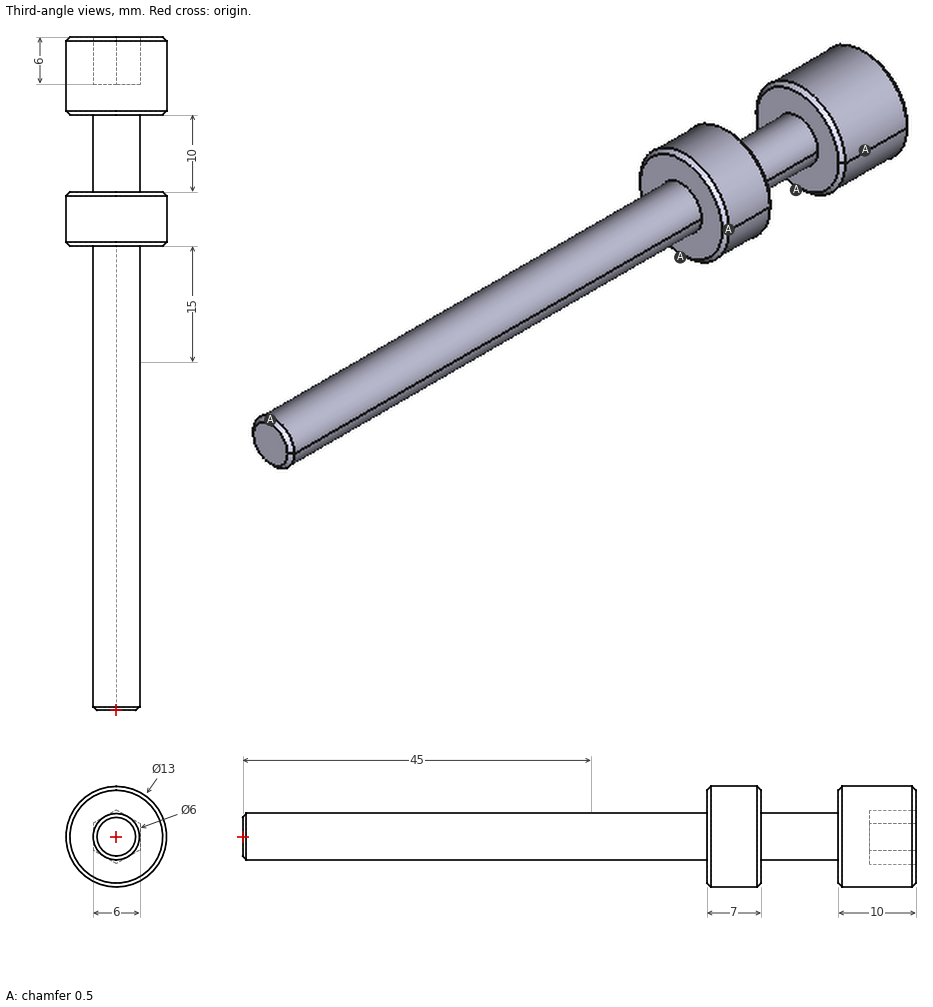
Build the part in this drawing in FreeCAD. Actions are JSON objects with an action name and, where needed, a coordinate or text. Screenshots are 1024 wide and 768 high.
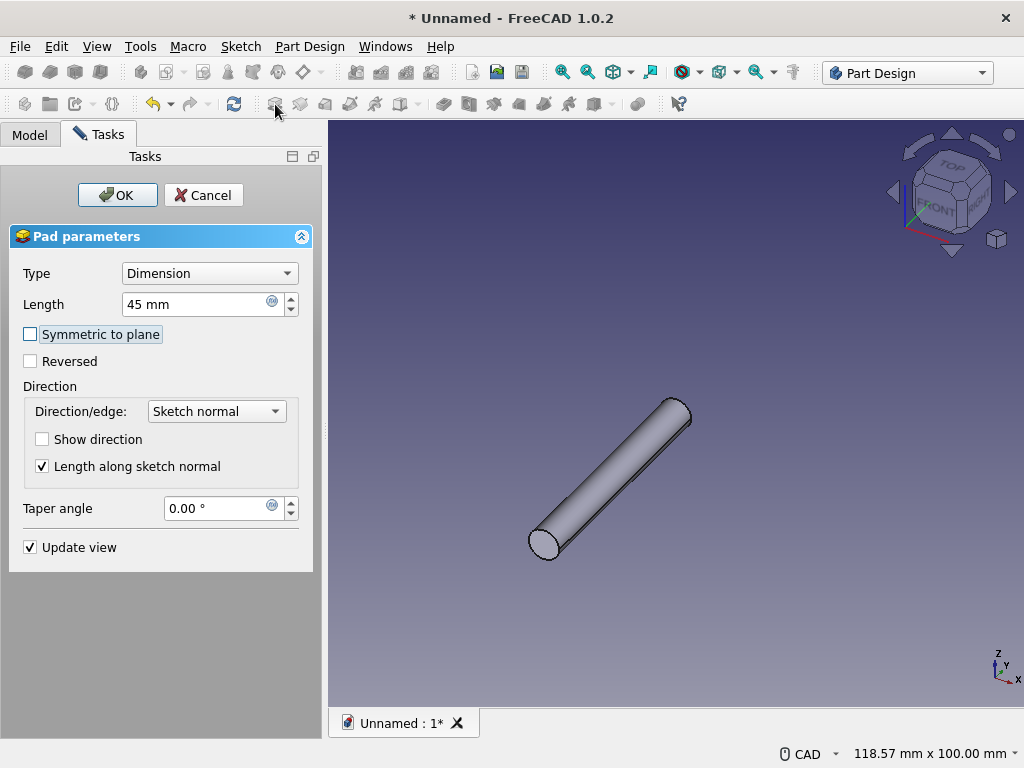
{"action": "left_click", "coordinate": [31, 361]}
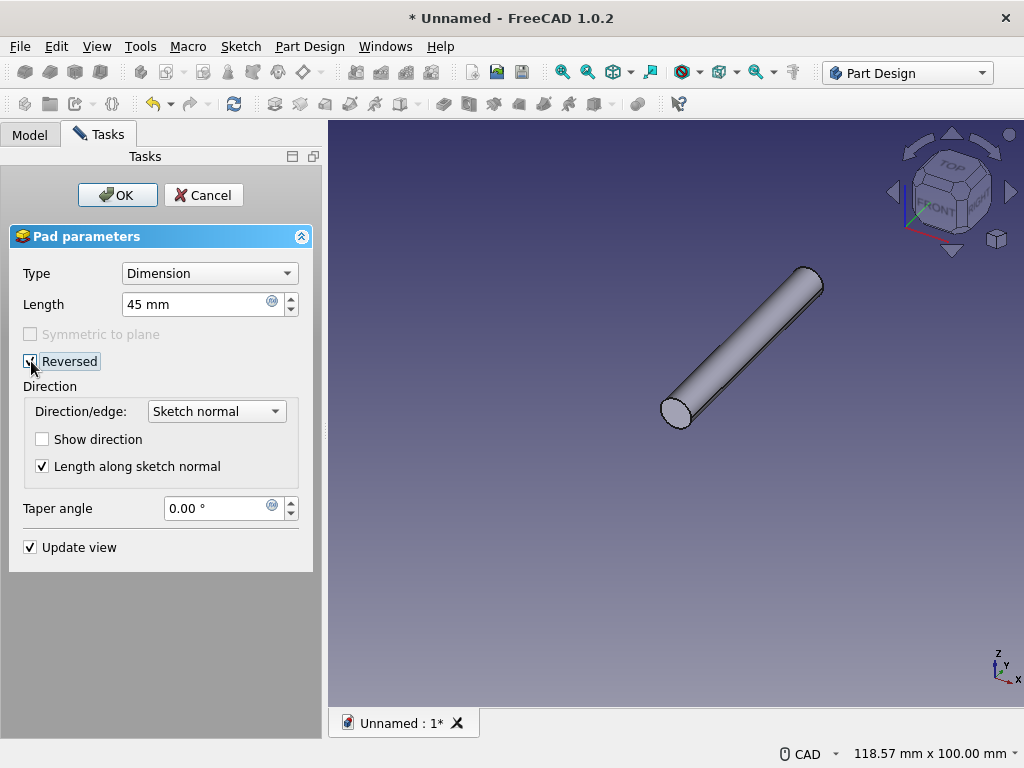
{"action": "left_click", "coordinate": [118, 195]}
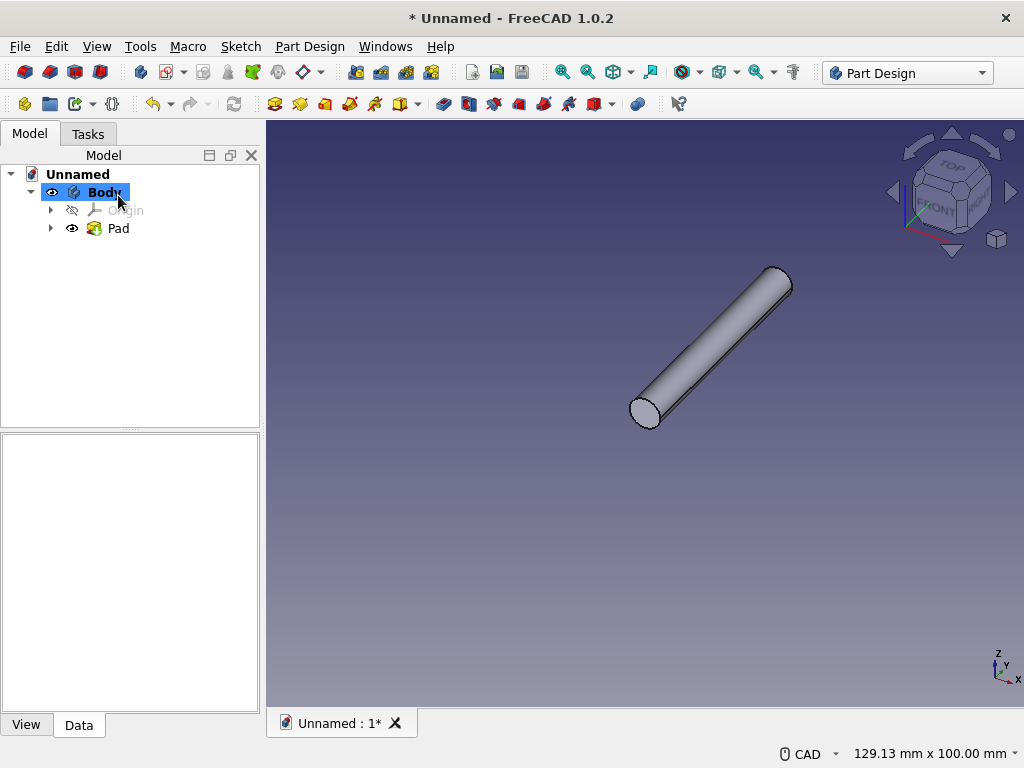
{"action": "left_click", "coordinate": [563, 72]}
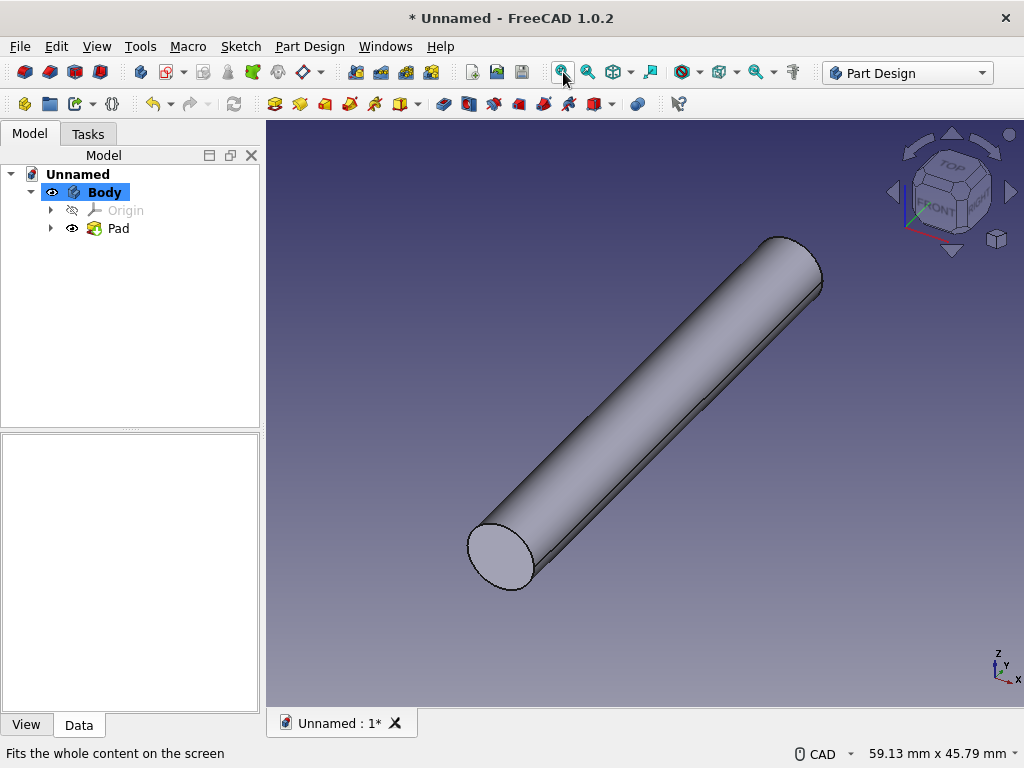
{"action": "key", "text": "4"}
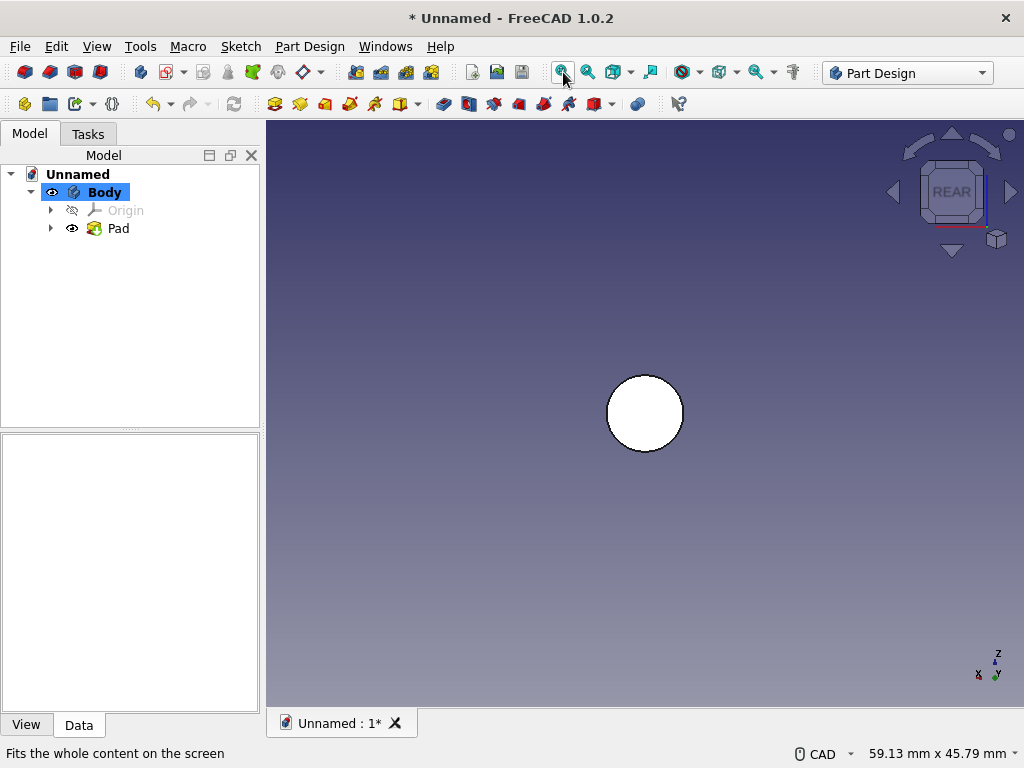
{"action": "left_click", "coordinate": [563, 72]}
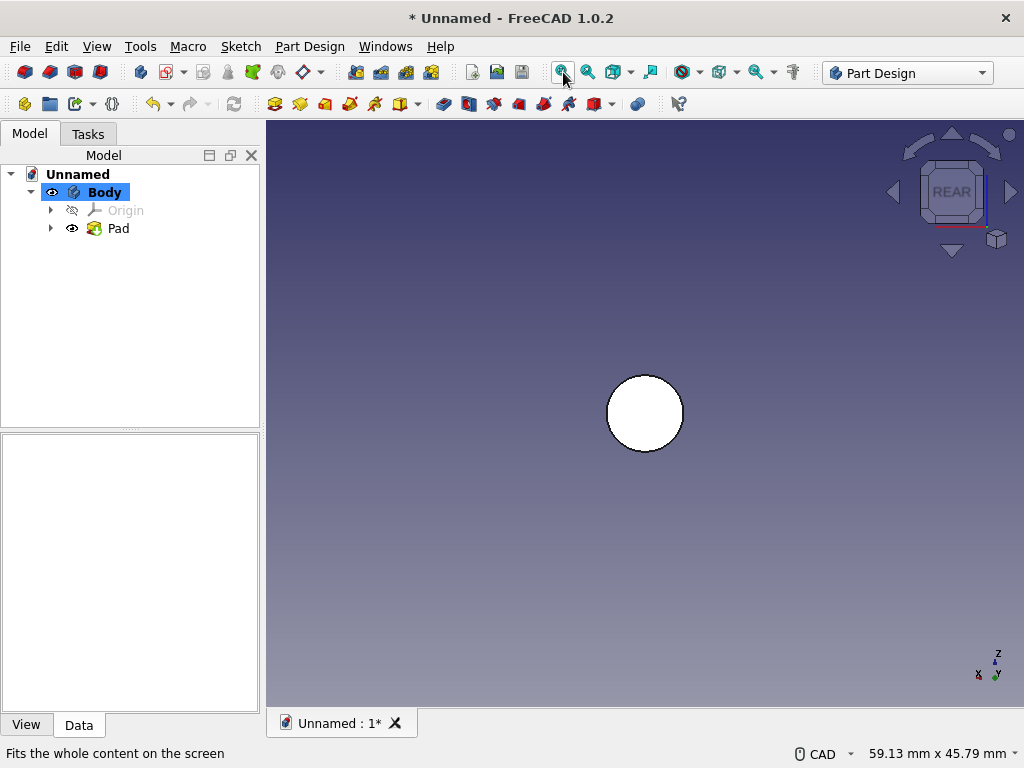
{"action": "left_click", "coordinate": [645, 413]}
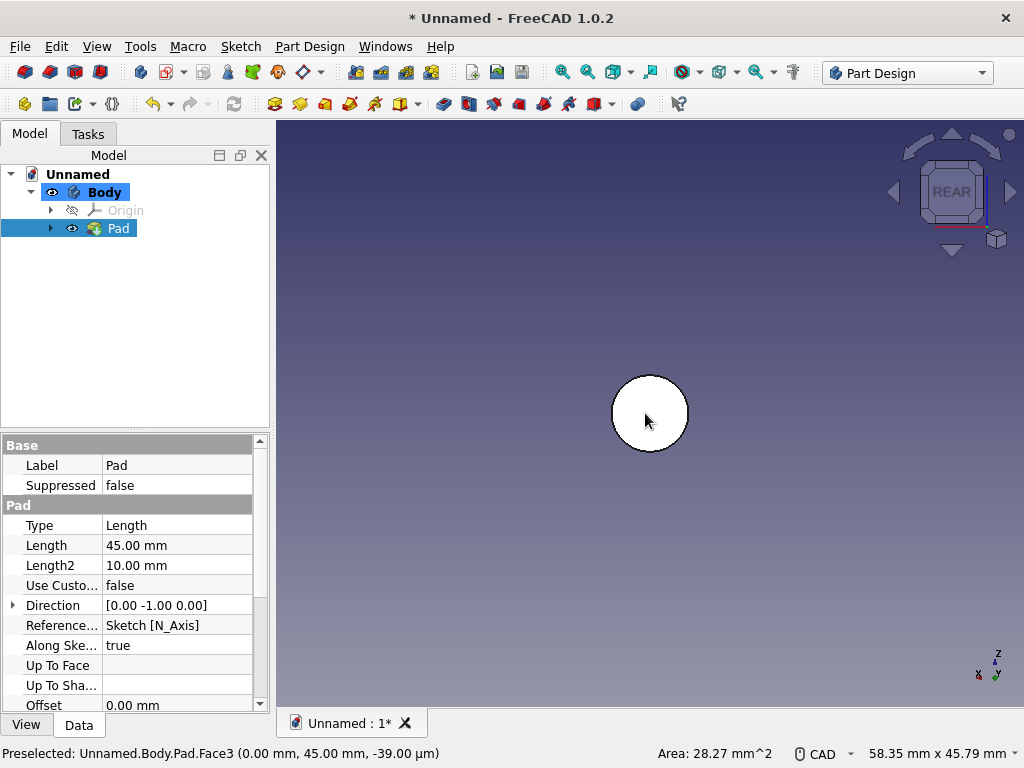
{"action": "left_click", "coordinate": [166, 72]}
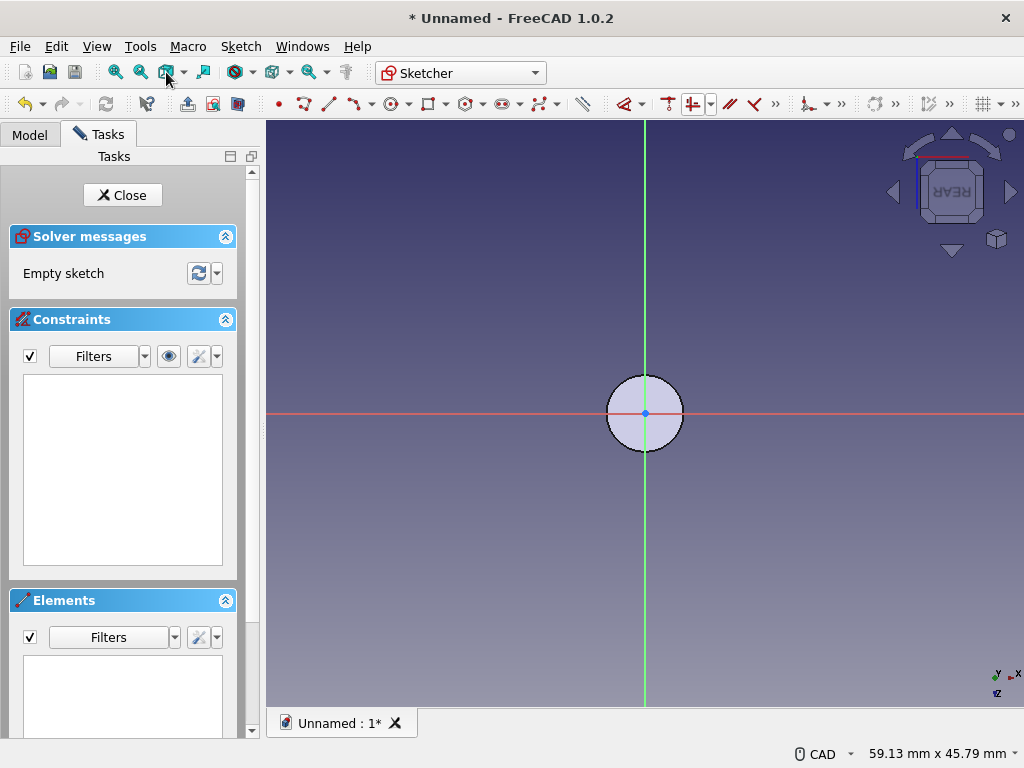
{"action": "scroll", "coordinate": [662, 413], "scroll_direction": "up", "scroll_amount": 8}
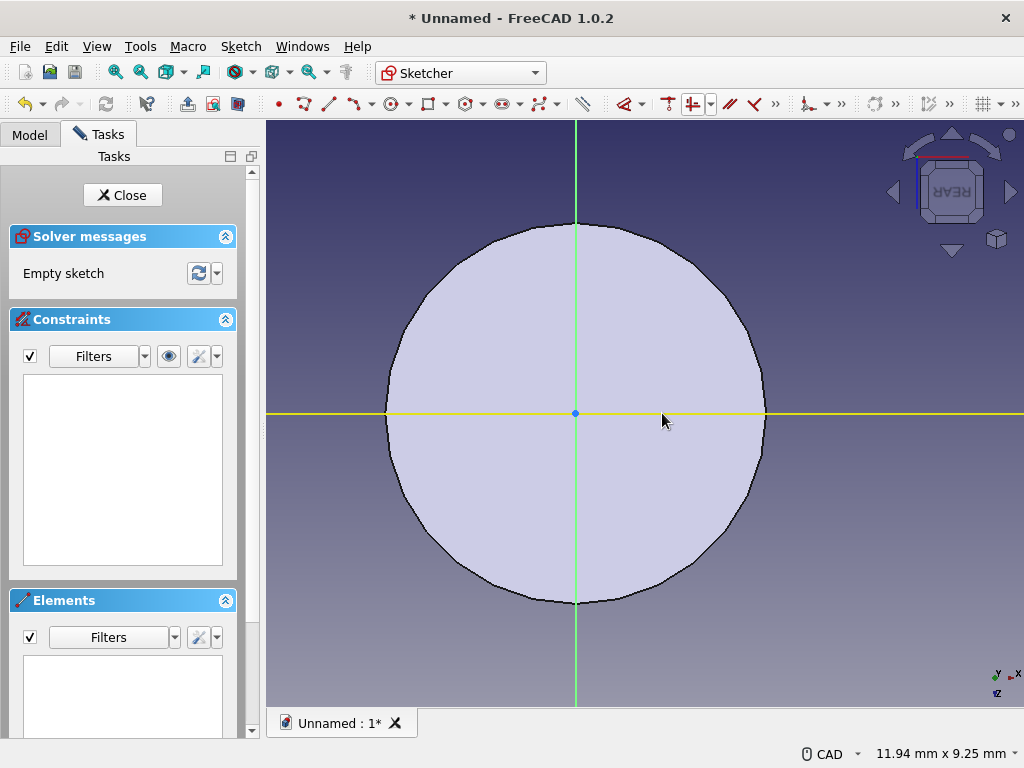
{"action": "left_click", "coordinate": [390, 104]}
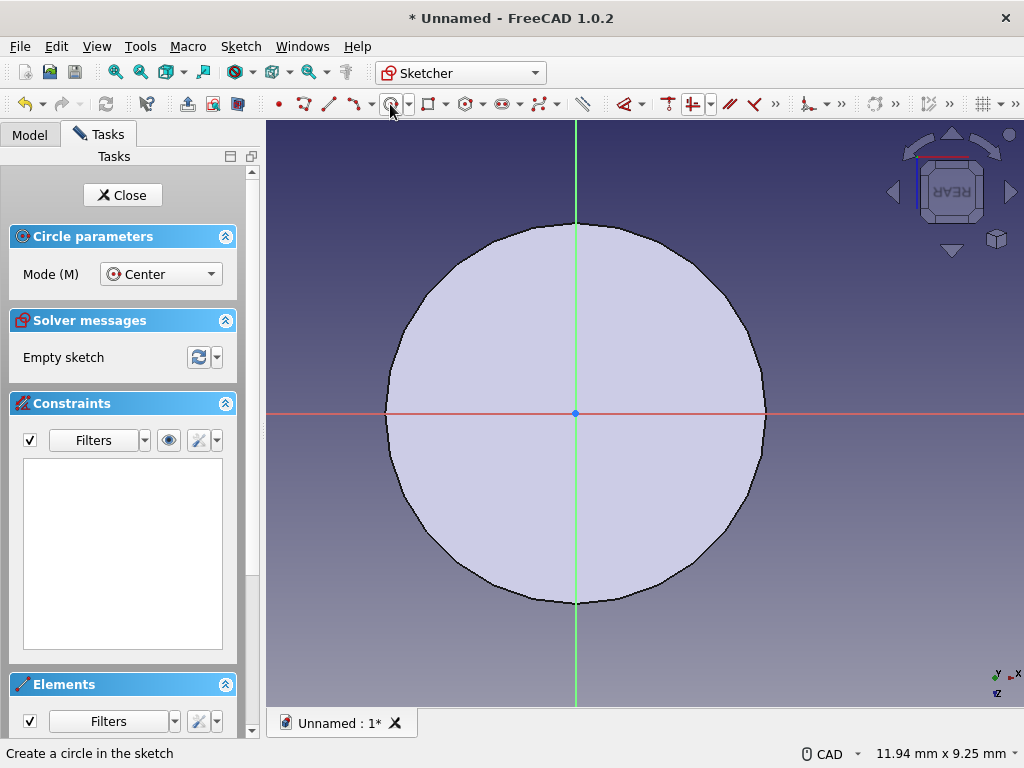
{"action": "left_click", "coordinate": [576, 413]}
{"action": "left_click", "coordinate": [710, 279]}
{"action": "key", "text": "Escape"}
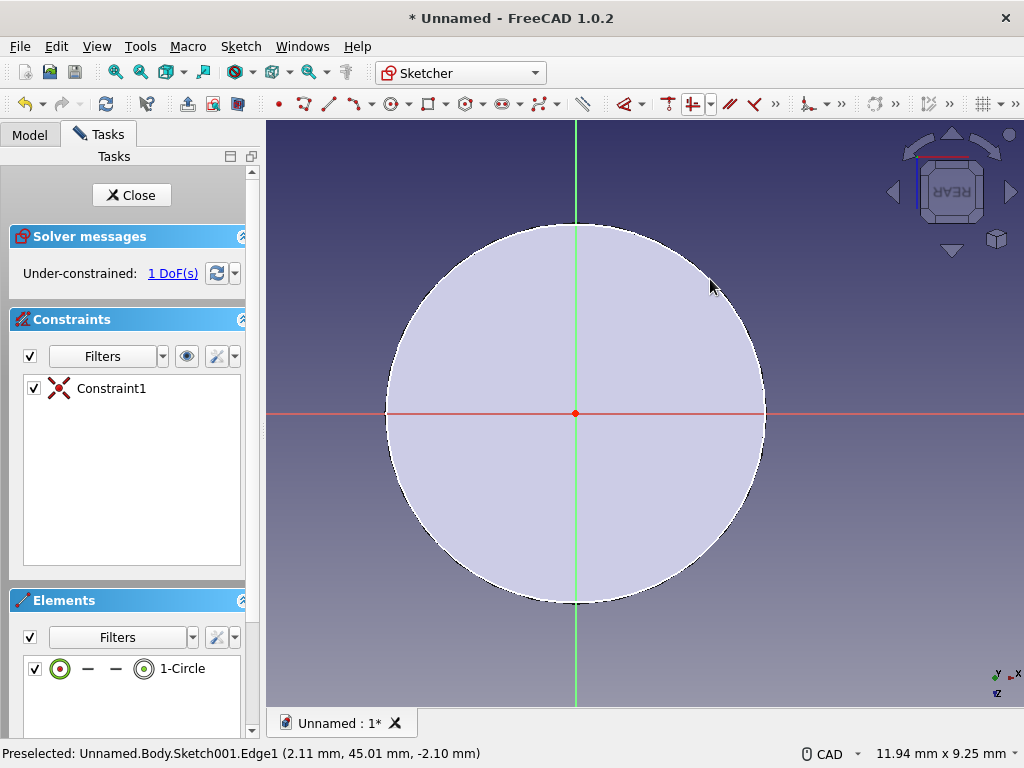
{"action": "left_click", "coordinate": [709, 279]}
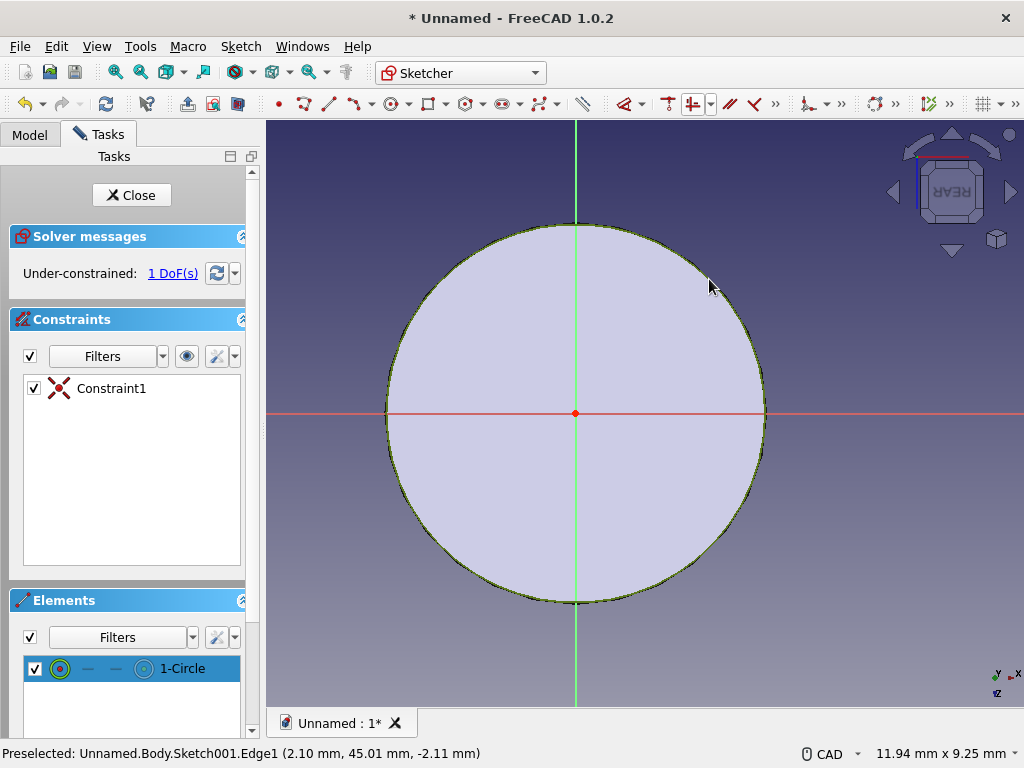
{"action": "left_click", "coordinate": [642, 104]}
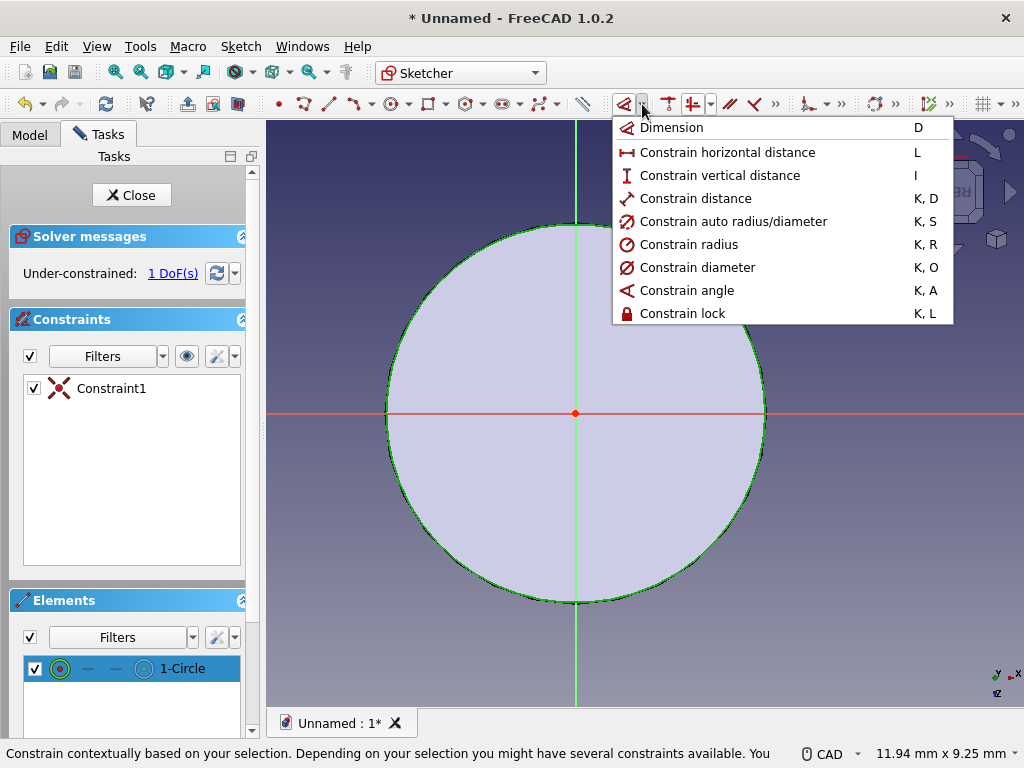
{"action": "left_click", "coordinate": [783, 268]}